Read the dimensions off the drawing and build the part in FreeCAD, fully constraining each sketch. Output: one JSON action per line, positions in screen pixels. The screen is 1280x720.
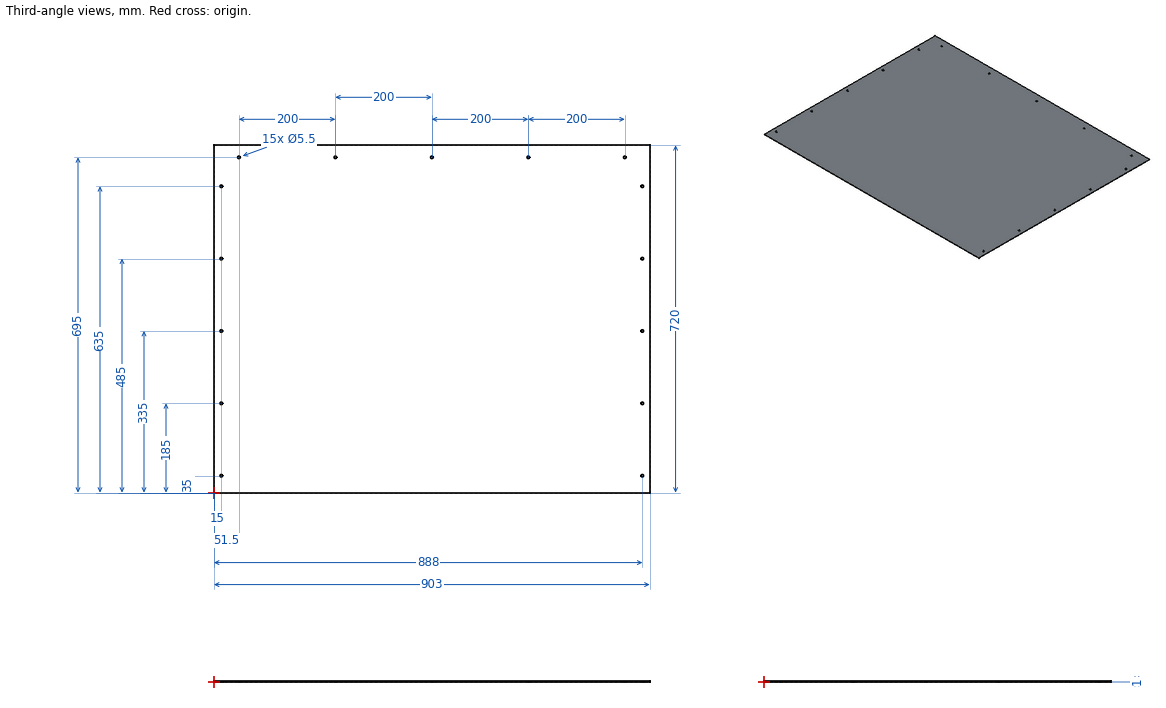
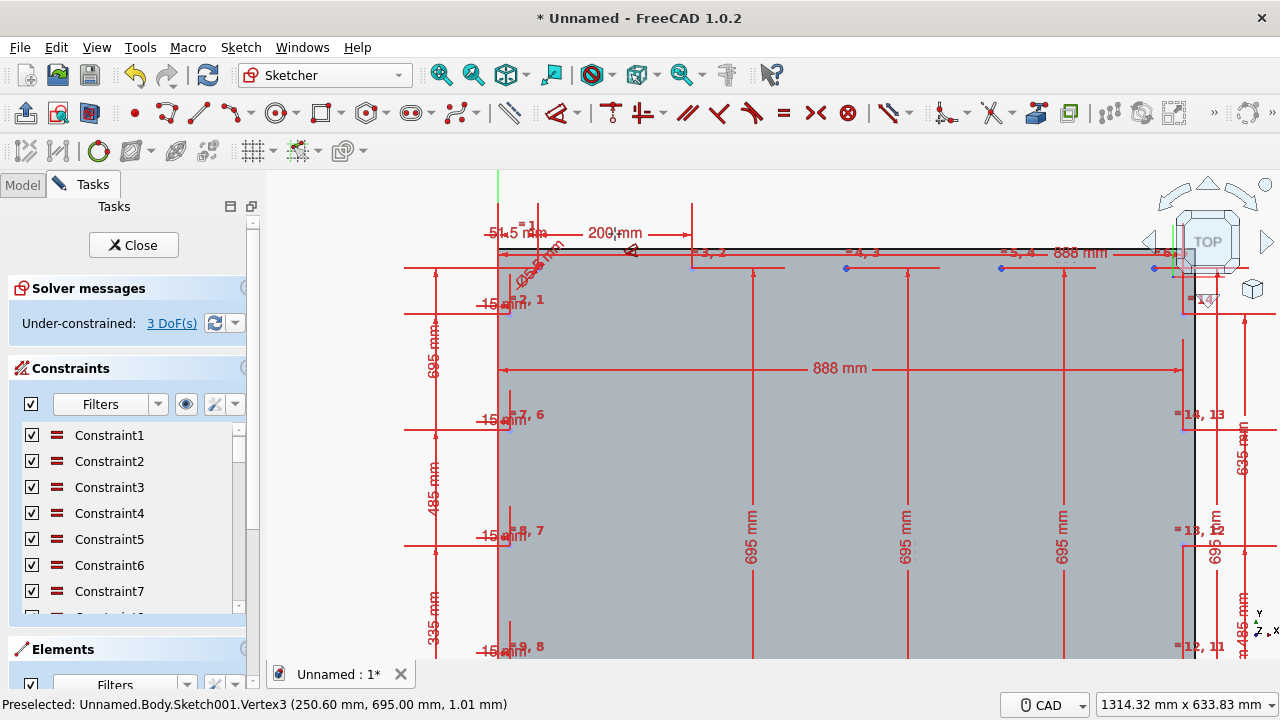
{"action": "left_click", "coordinate": [692, 268]}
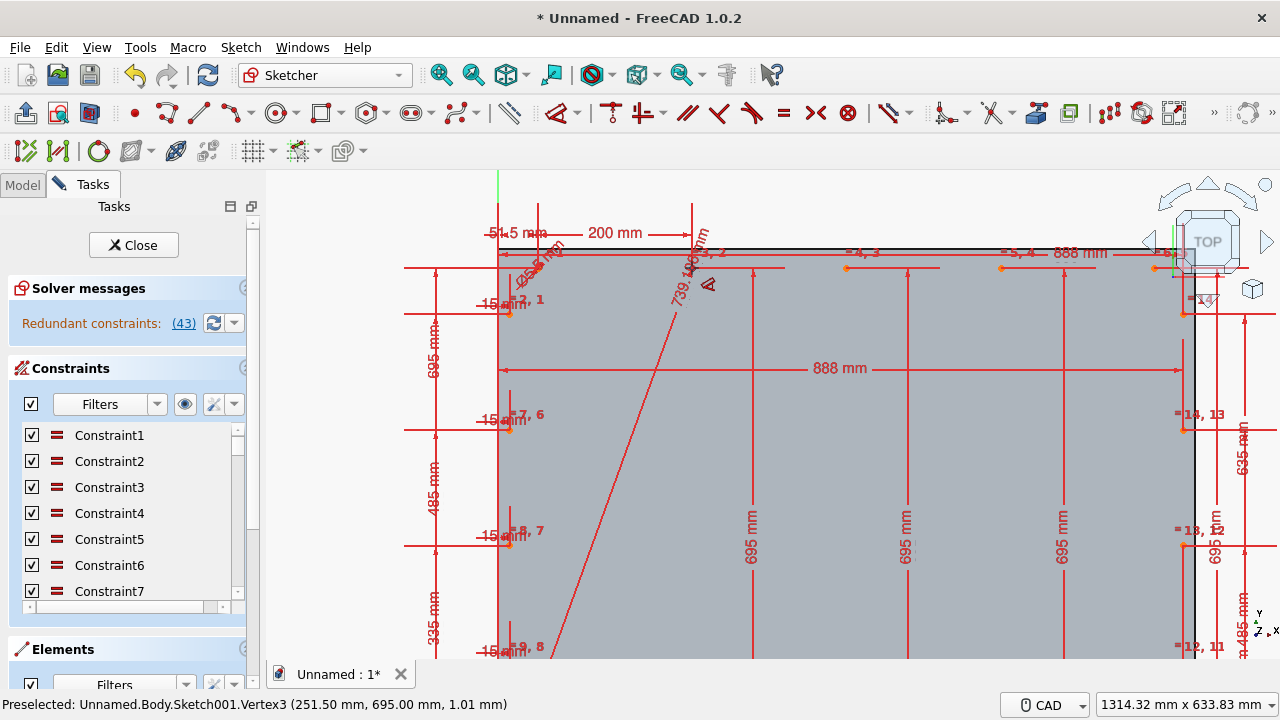
{"action": "left_click", "coordinate": [847, 268]}
{"action": "left_click", "coordinate": [769, 234]}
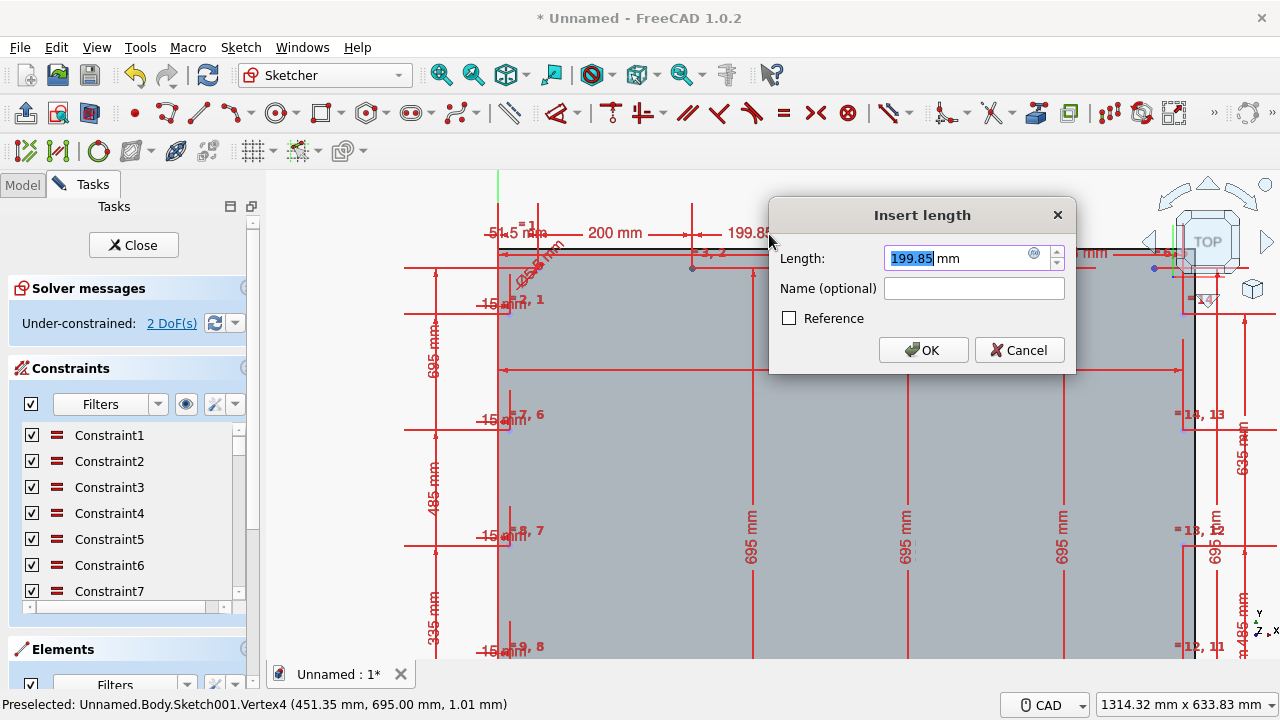
{"action": "type", "text": "200"}
{"action": "key", "text": "Return"}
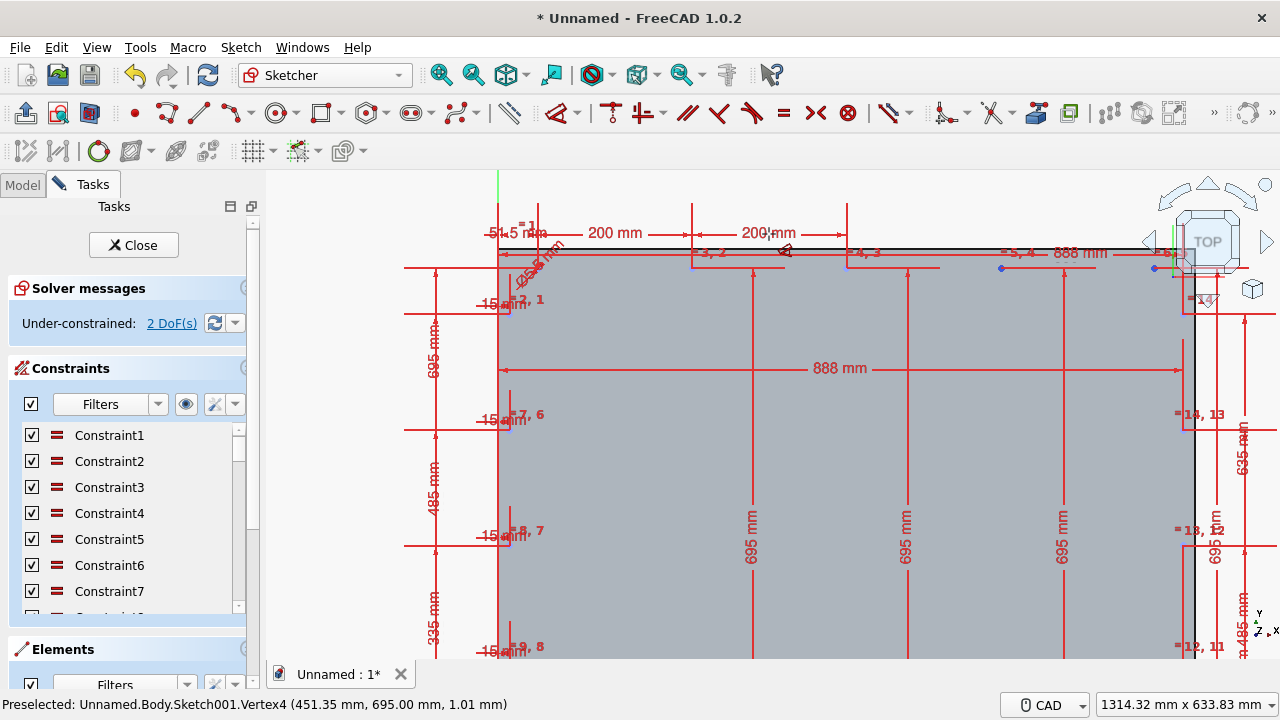
{"action": "left_click", "coordinate": [847, 268]}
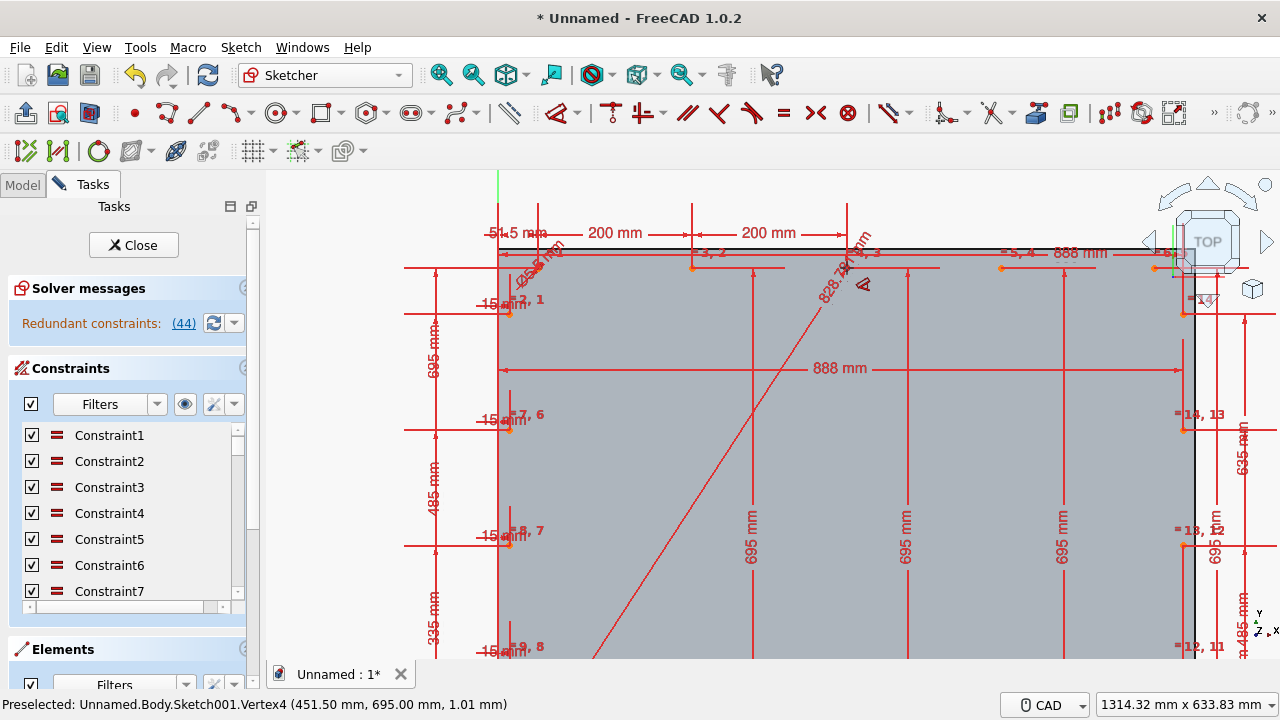
{"action": "left_click", "coordinate": [1002, 268]}
{"action": "left_click", "coordinate": [924, 234]}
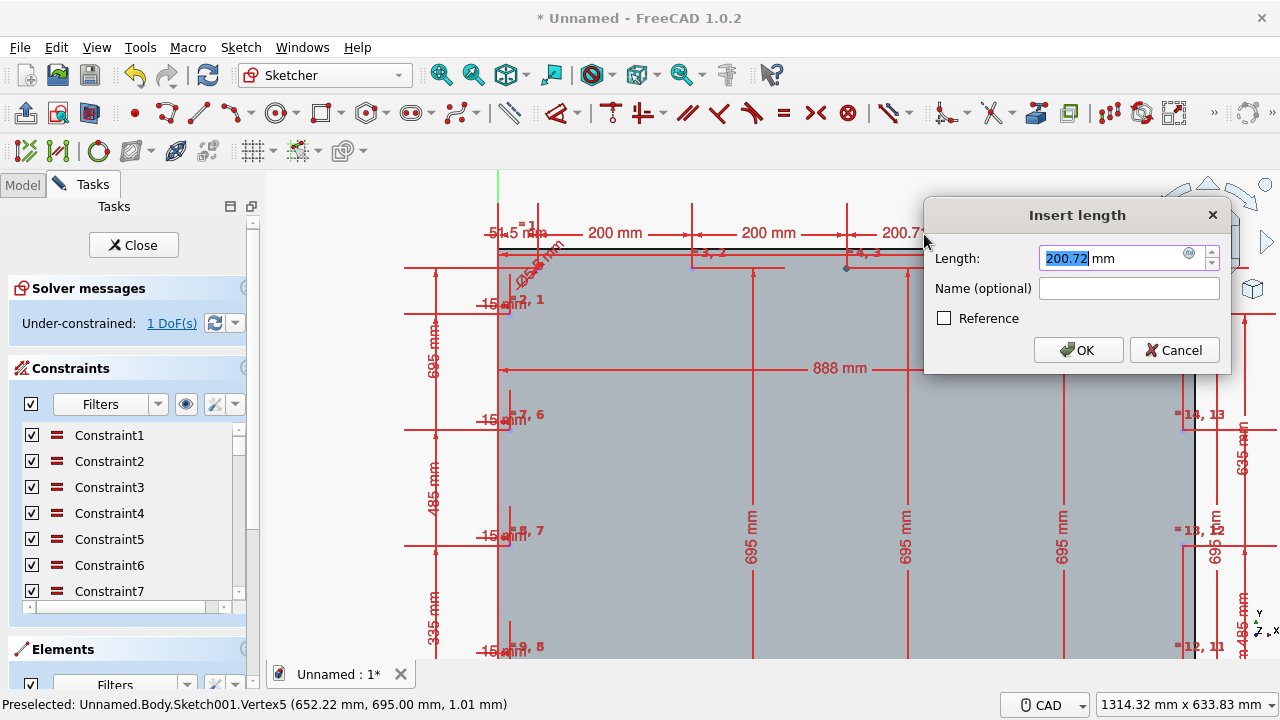
{"action": "type", "text": "200"}
{"action": "key", "text": "Return"}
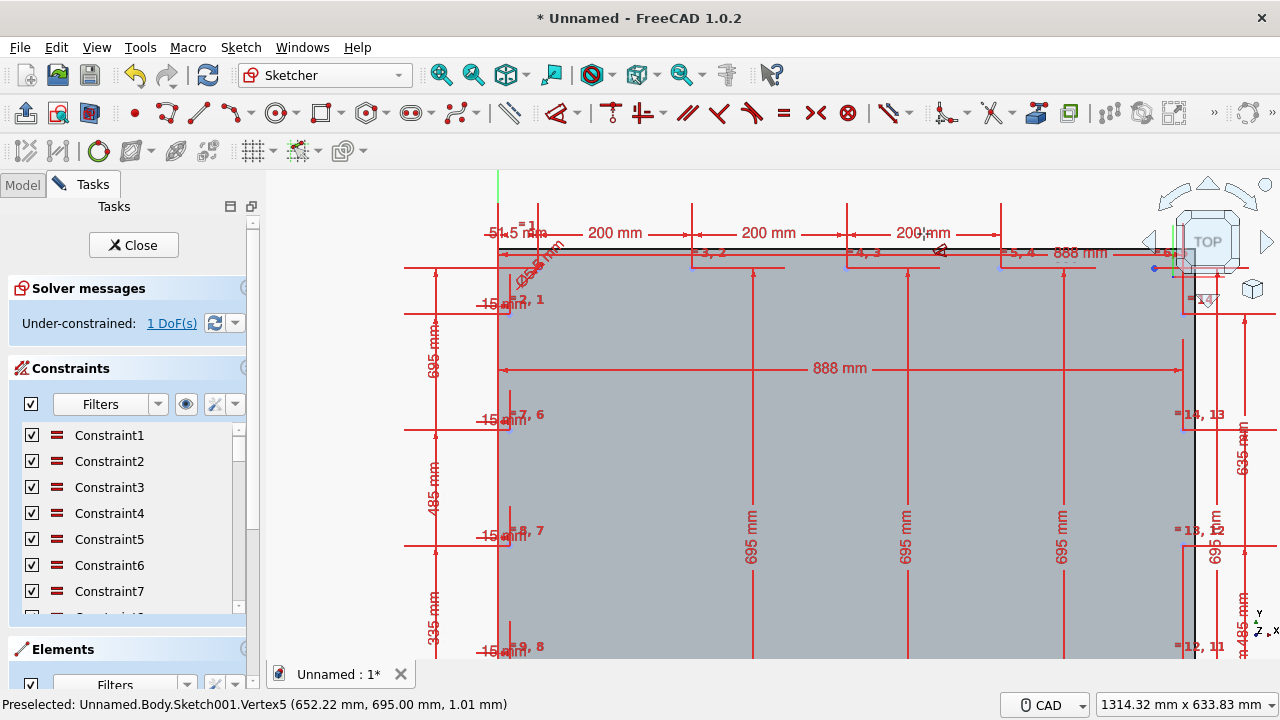
{"action": "left_click", "coordinate": [1001, 268]}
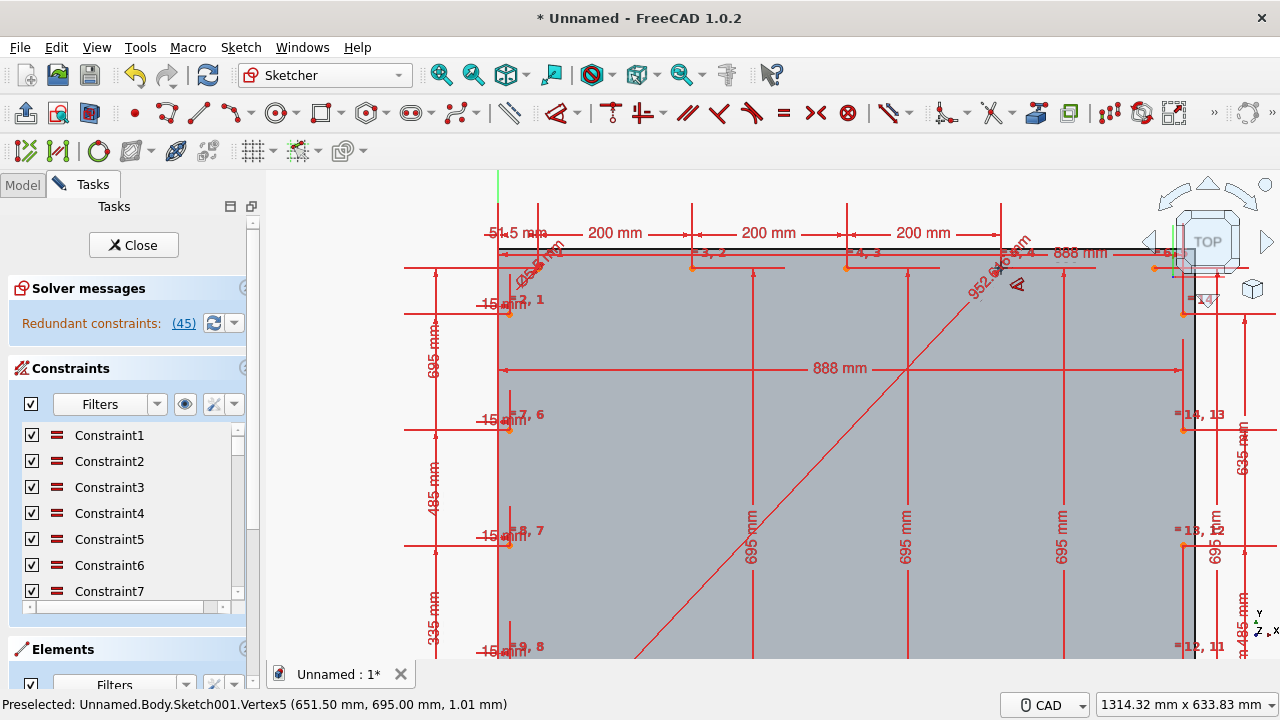
{"action": "scroll", "coordinate": [537, 268], "scroll_direction": "down", "scroll_amount": 3}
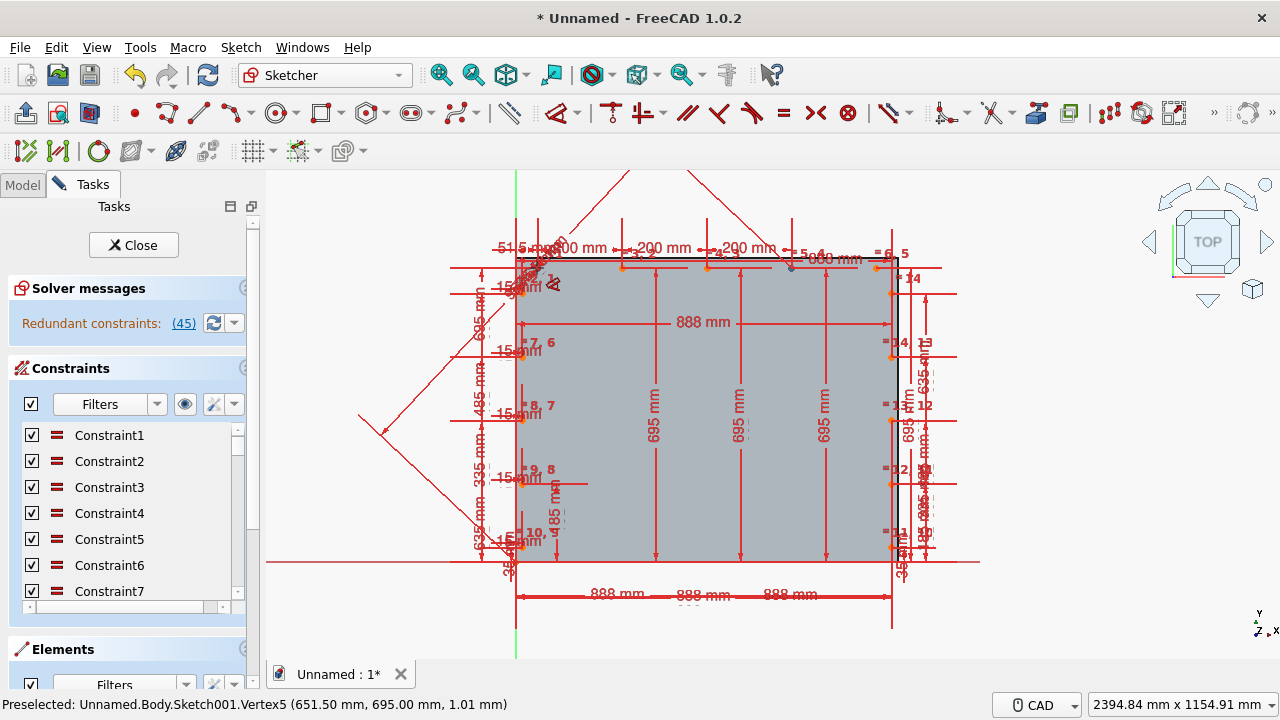
{"action": "left_click", "coordinate": [876, 268]}
{"action": "left_click", "coordinate": [834, 234]}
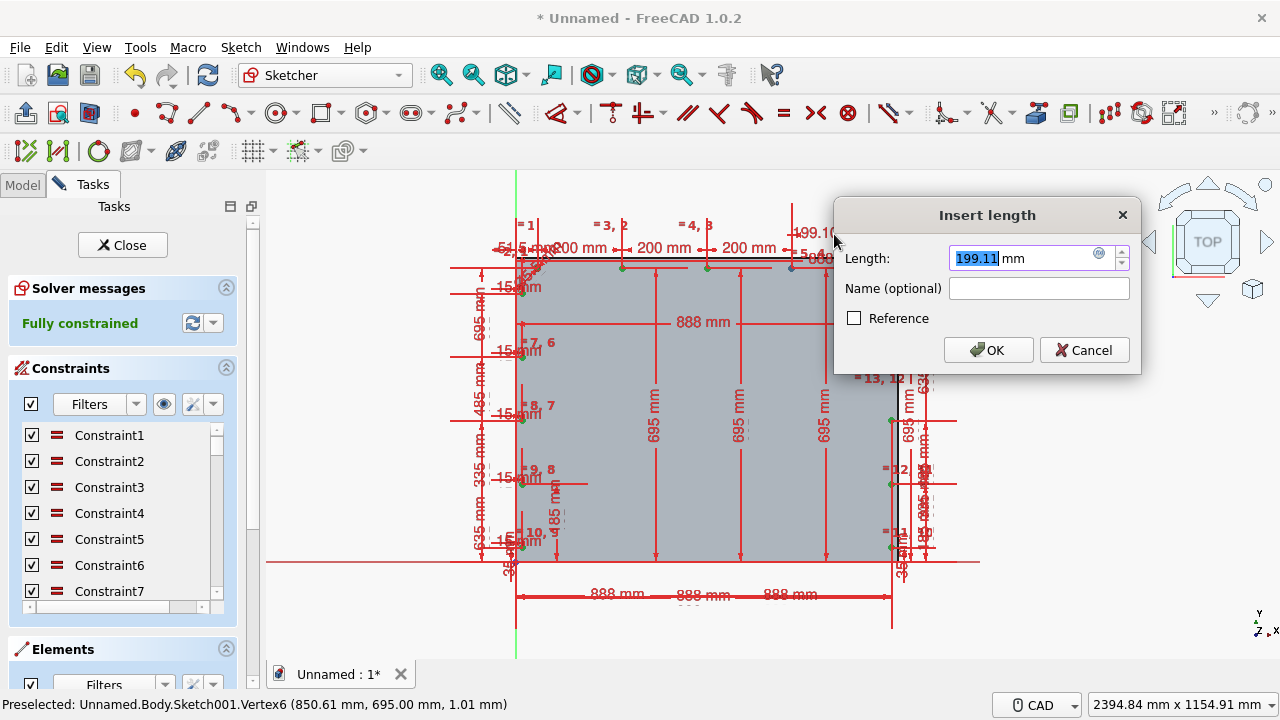
{"action": "type", "text": "200"}
{"action": "key", "text": "Return"}
{"action": "key", "text": "Escape"}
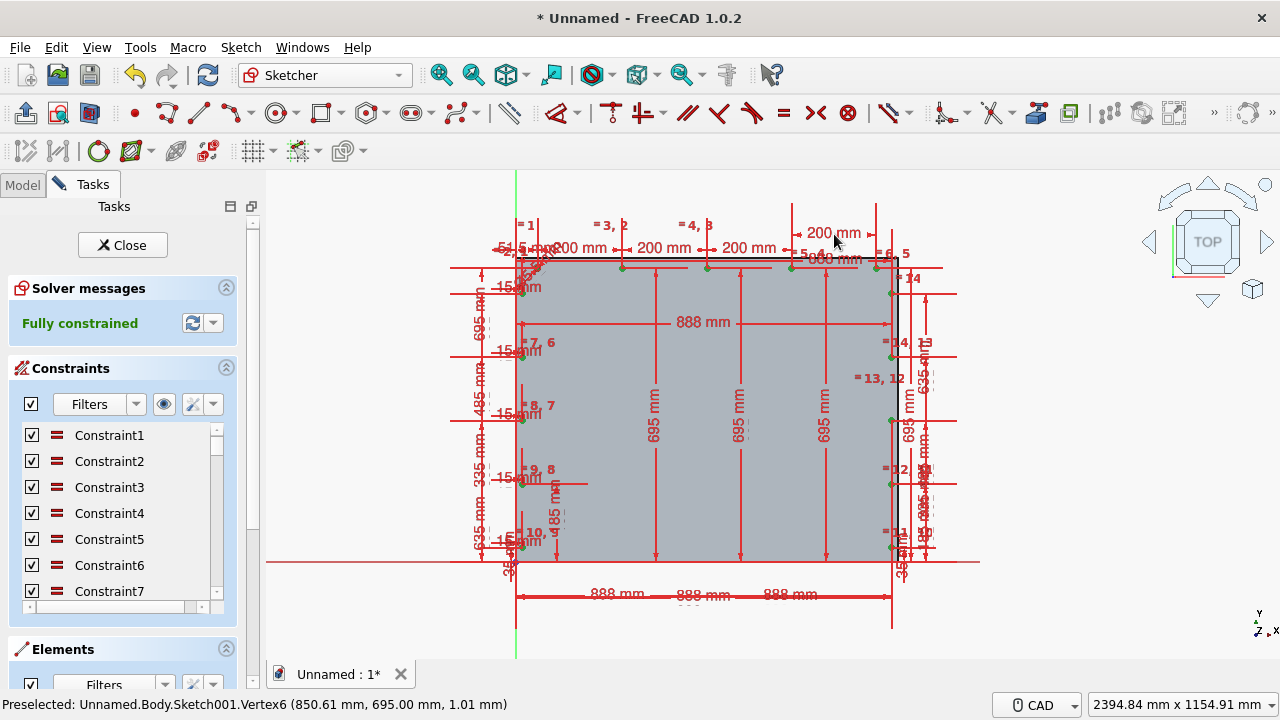
{"action": "left_click", "coordinate": [123, 245]}